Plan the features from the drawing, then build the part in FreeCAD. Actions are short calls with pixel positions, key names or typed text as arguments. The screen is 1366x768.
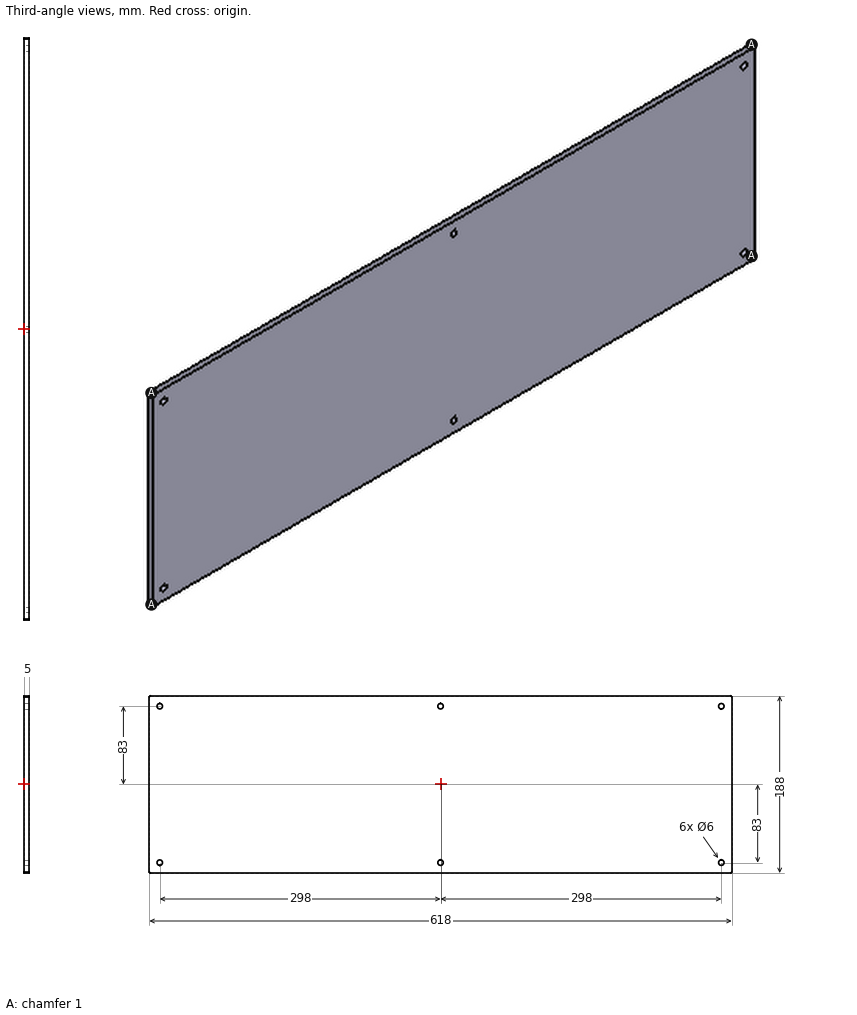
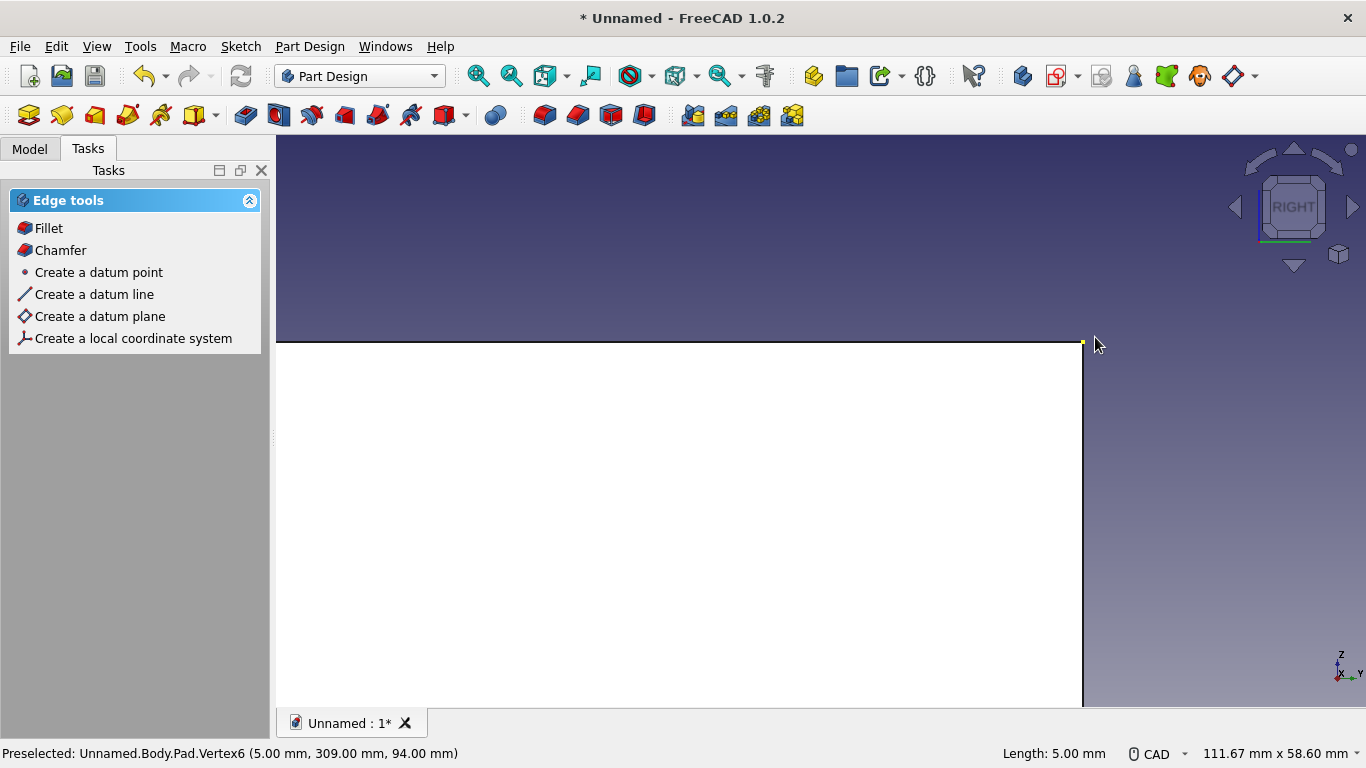
click(479, 76)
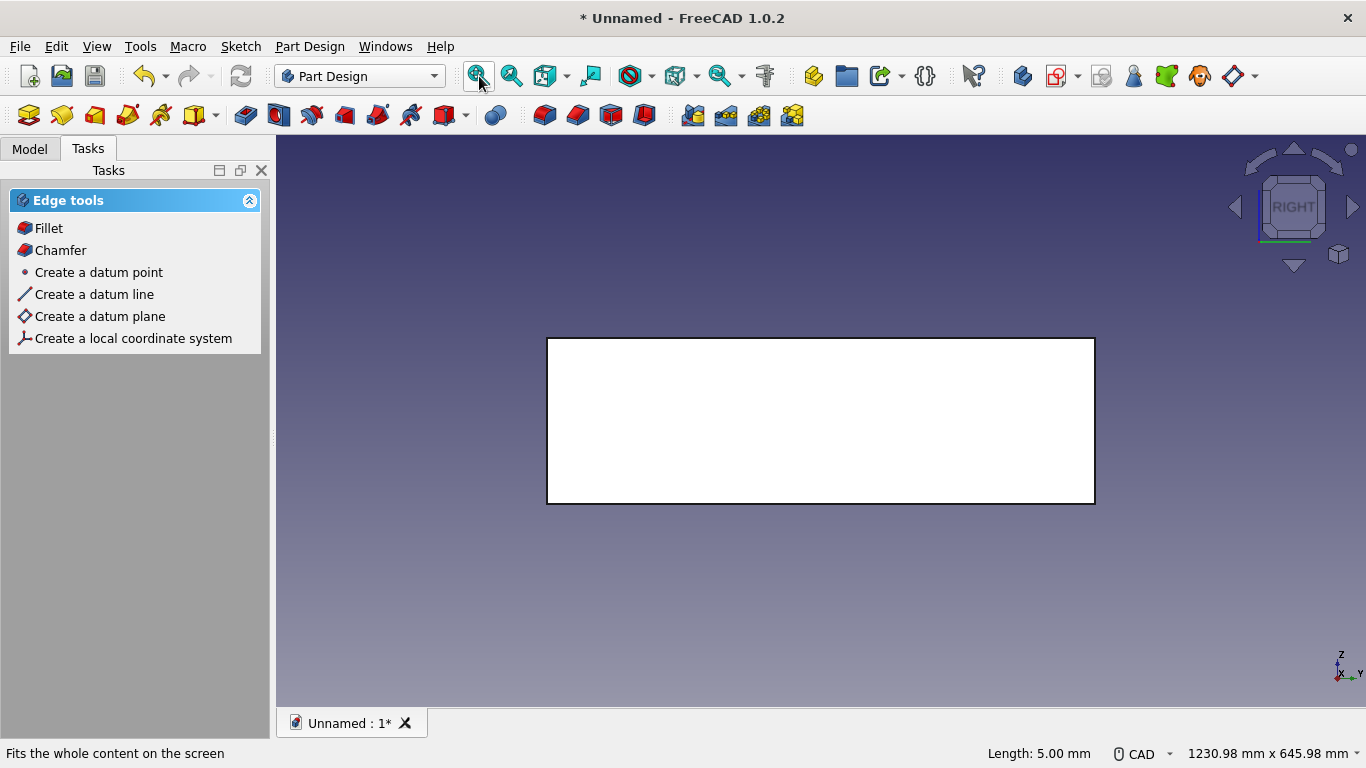
key(5)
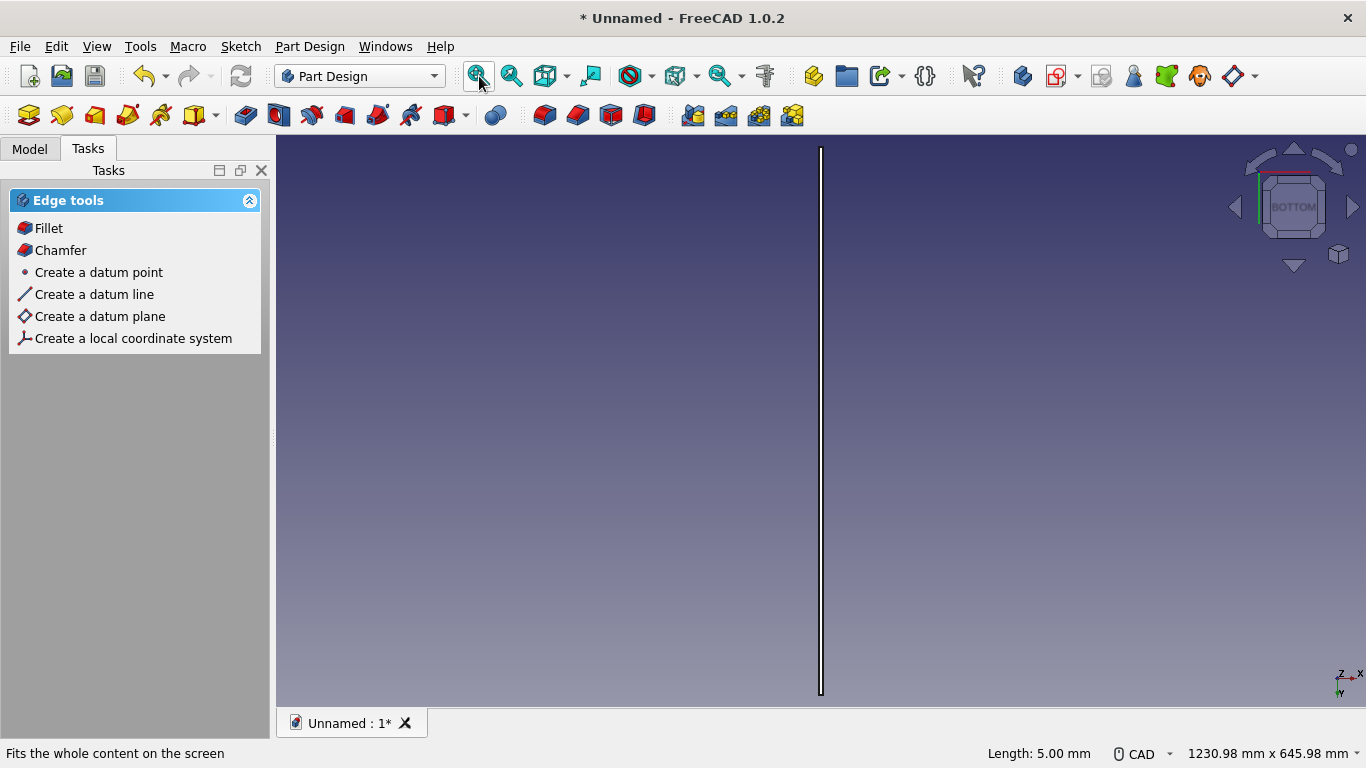
key(4)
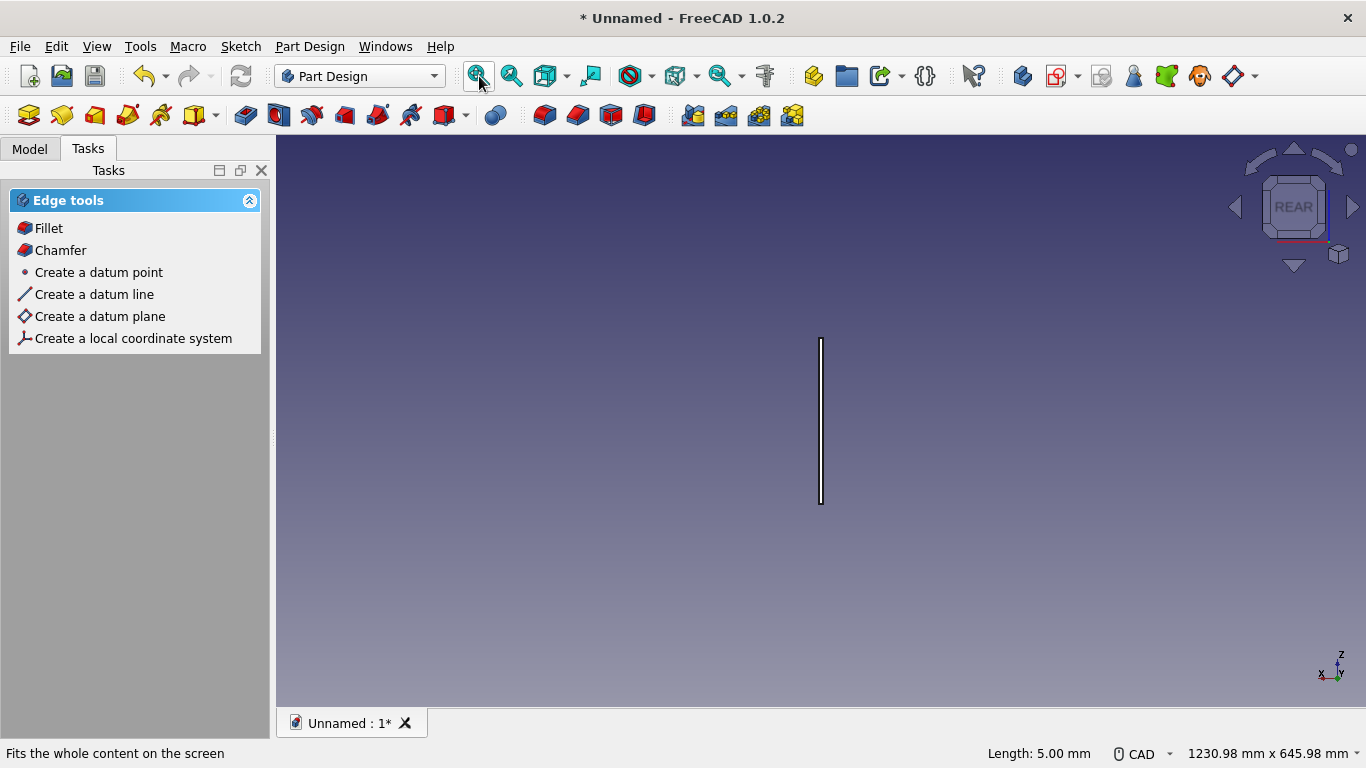
click(479, 76)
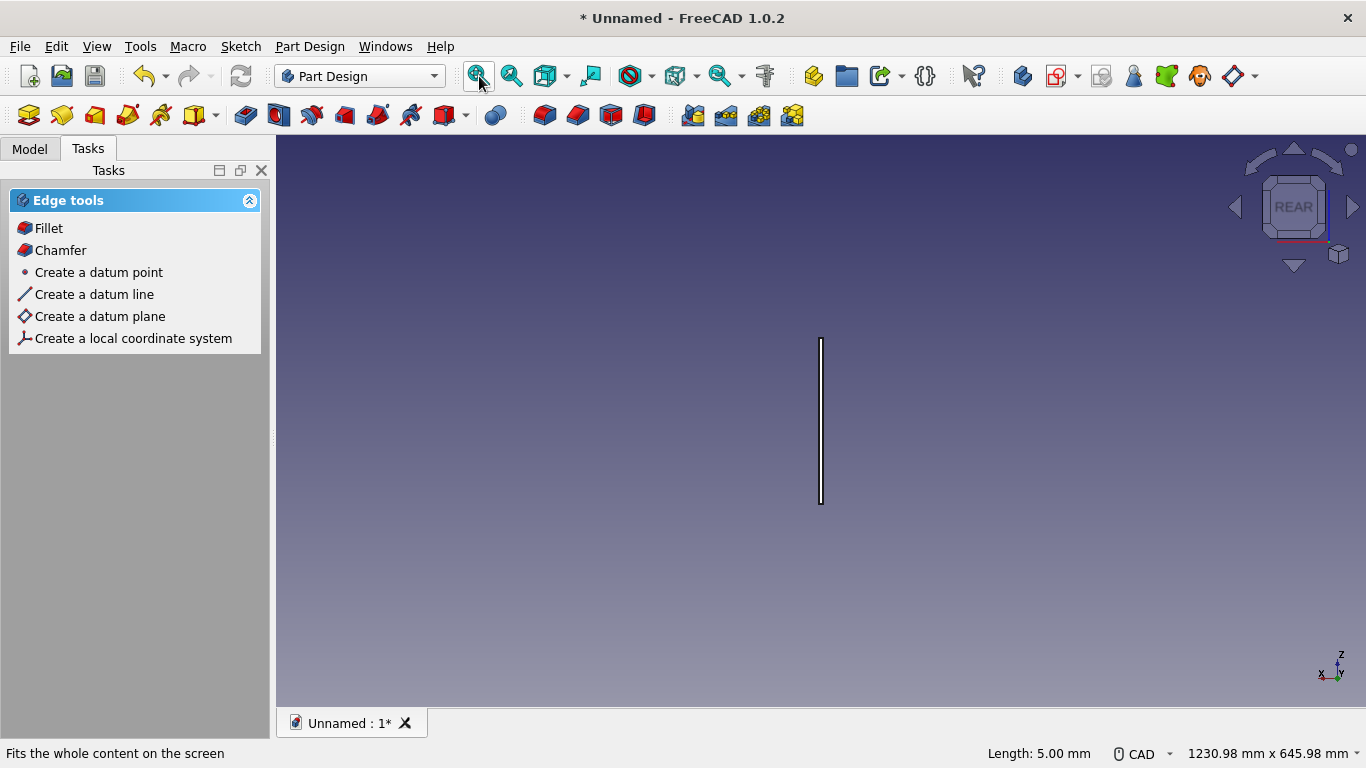
scroll(821, 337, up, 12)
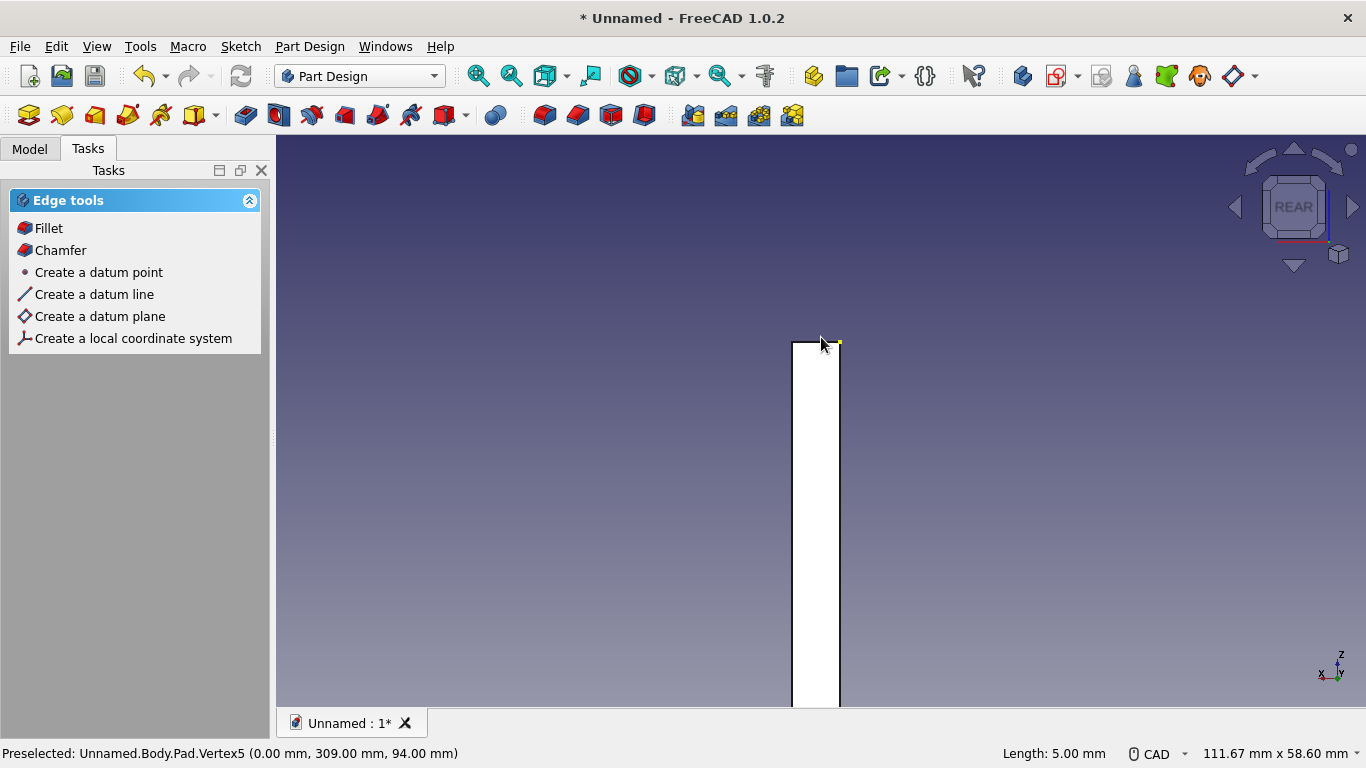
click(816, 341, ctrl)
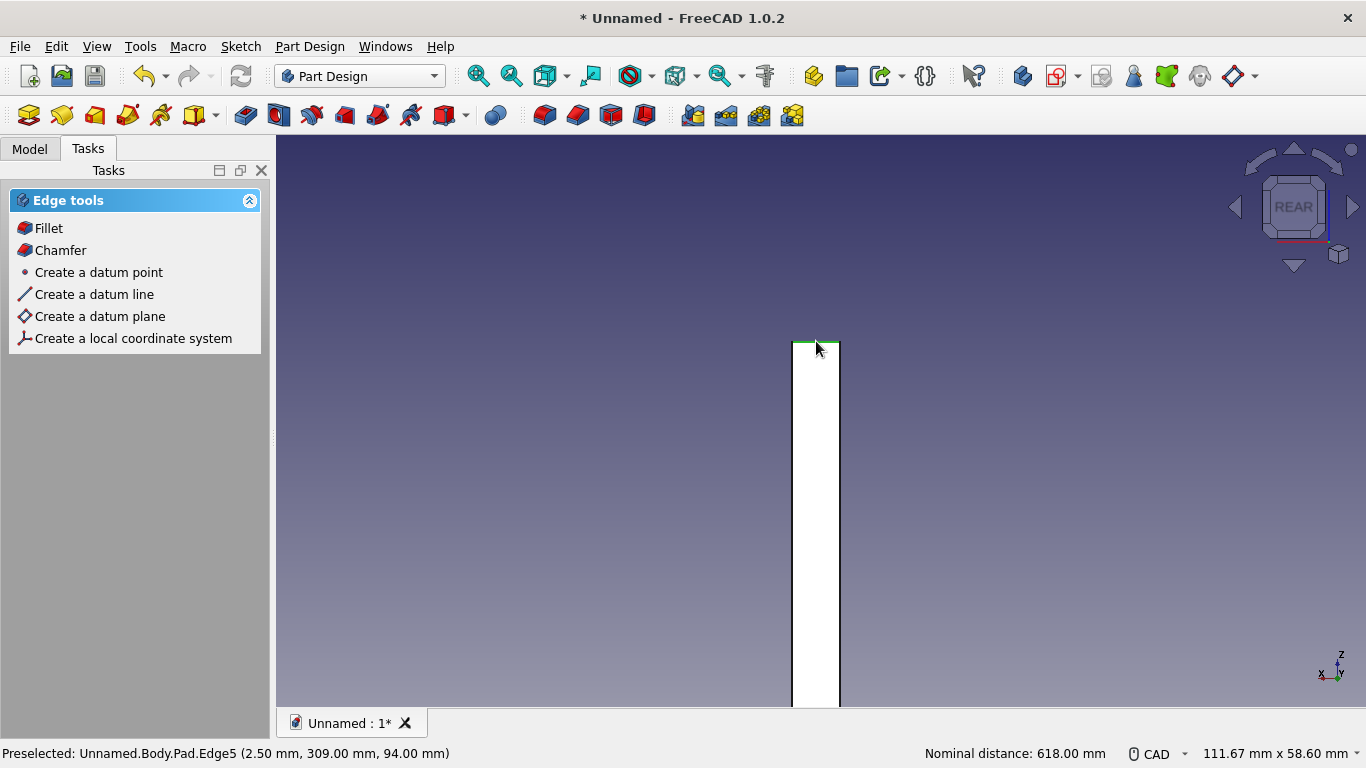
click(479, 76)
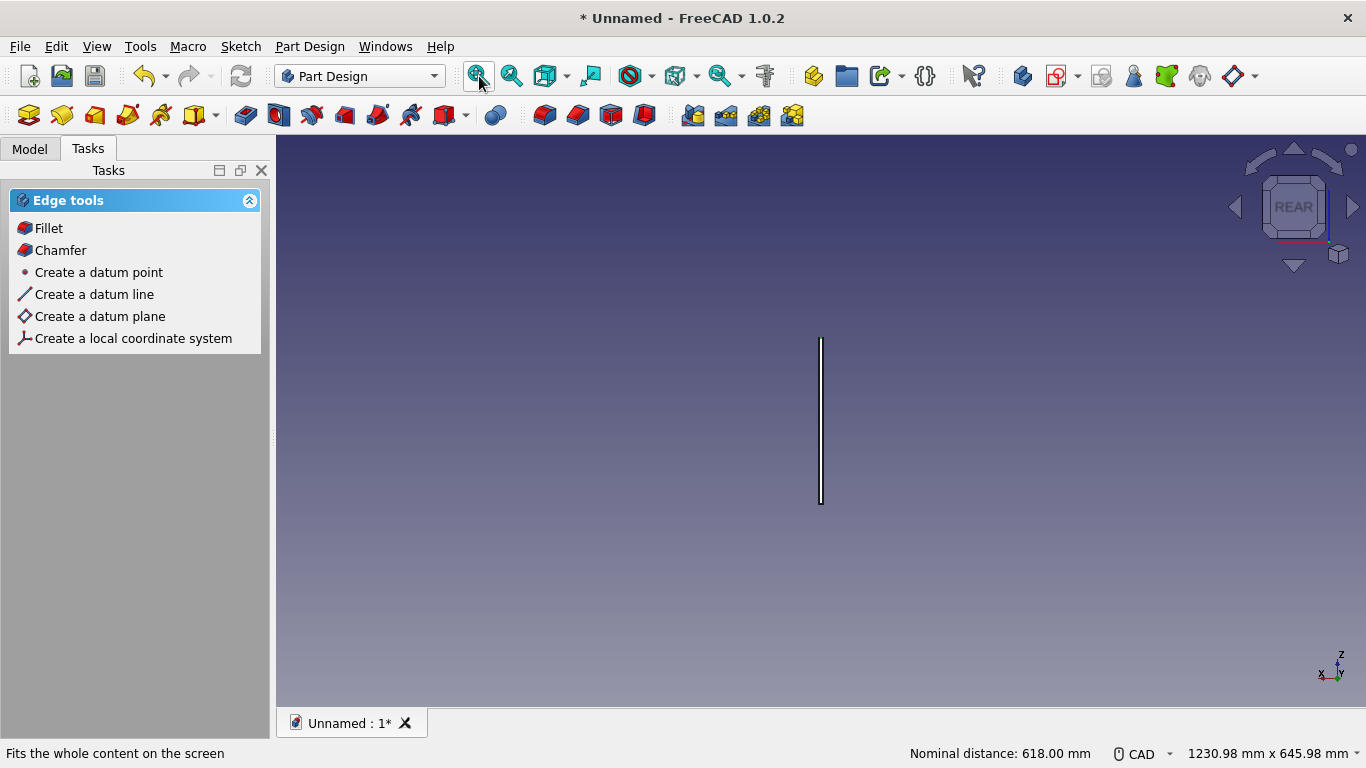
key(6)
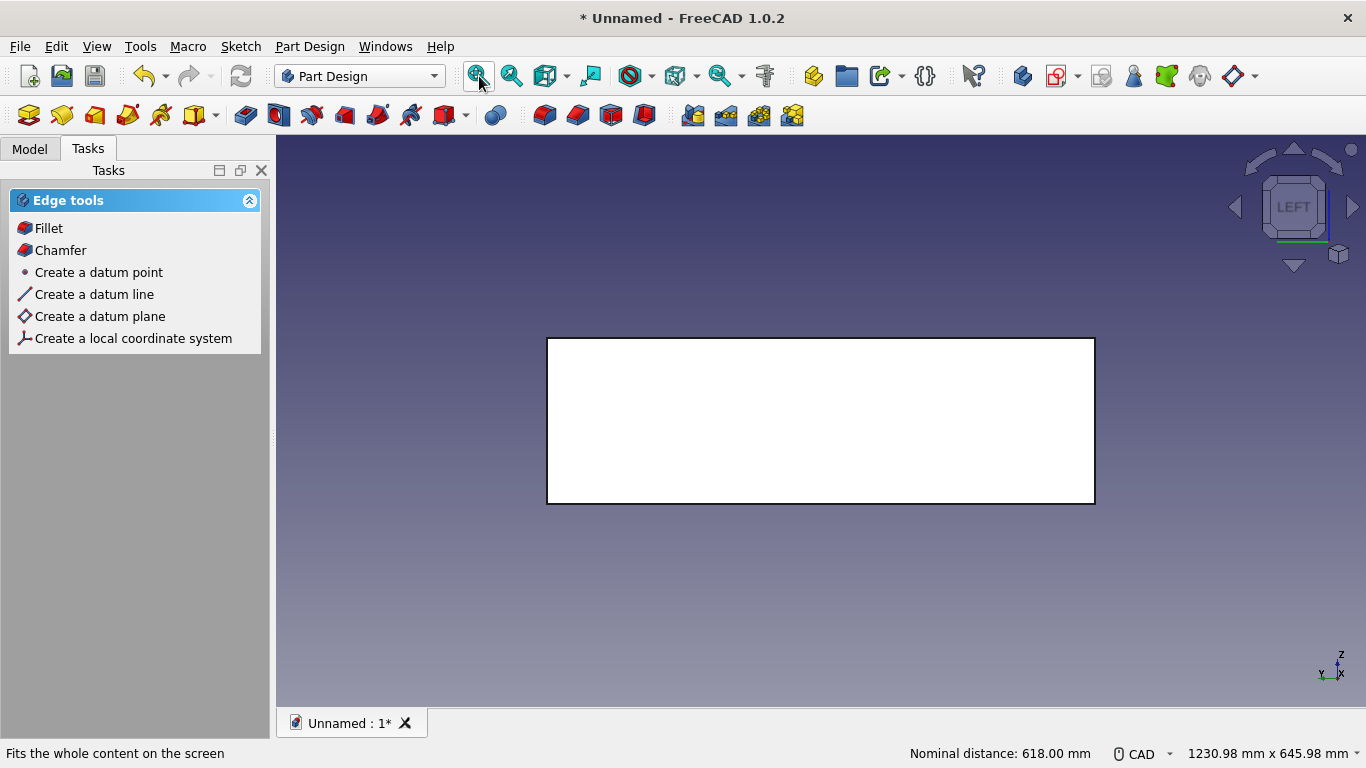
scroll(547, 503, up, 12)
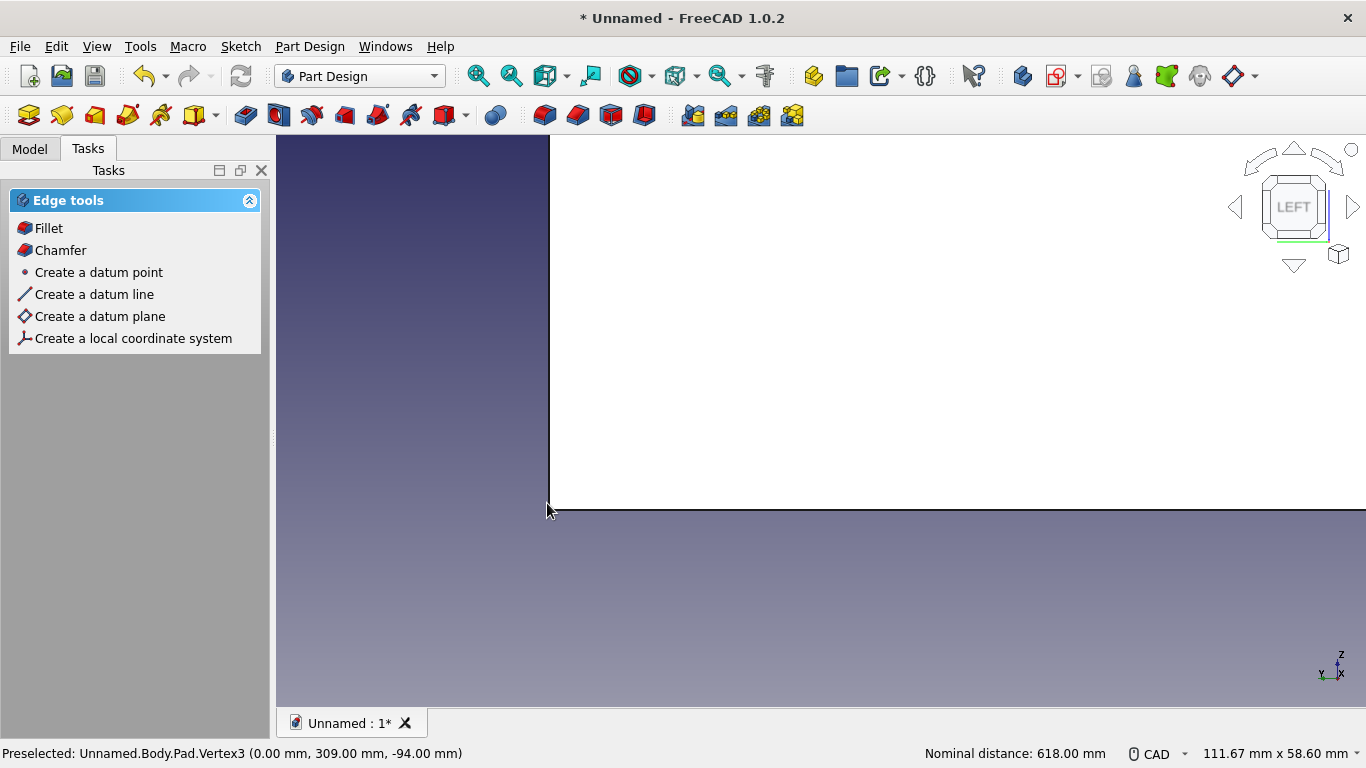
click(479, 76)